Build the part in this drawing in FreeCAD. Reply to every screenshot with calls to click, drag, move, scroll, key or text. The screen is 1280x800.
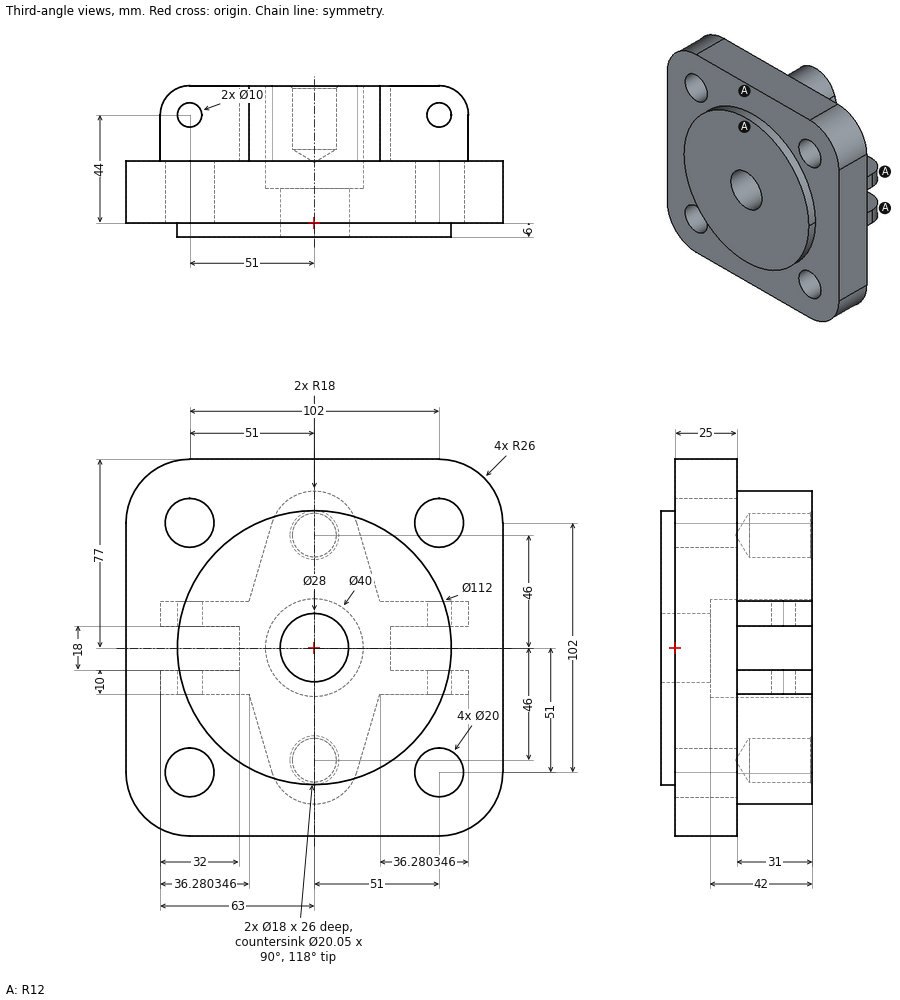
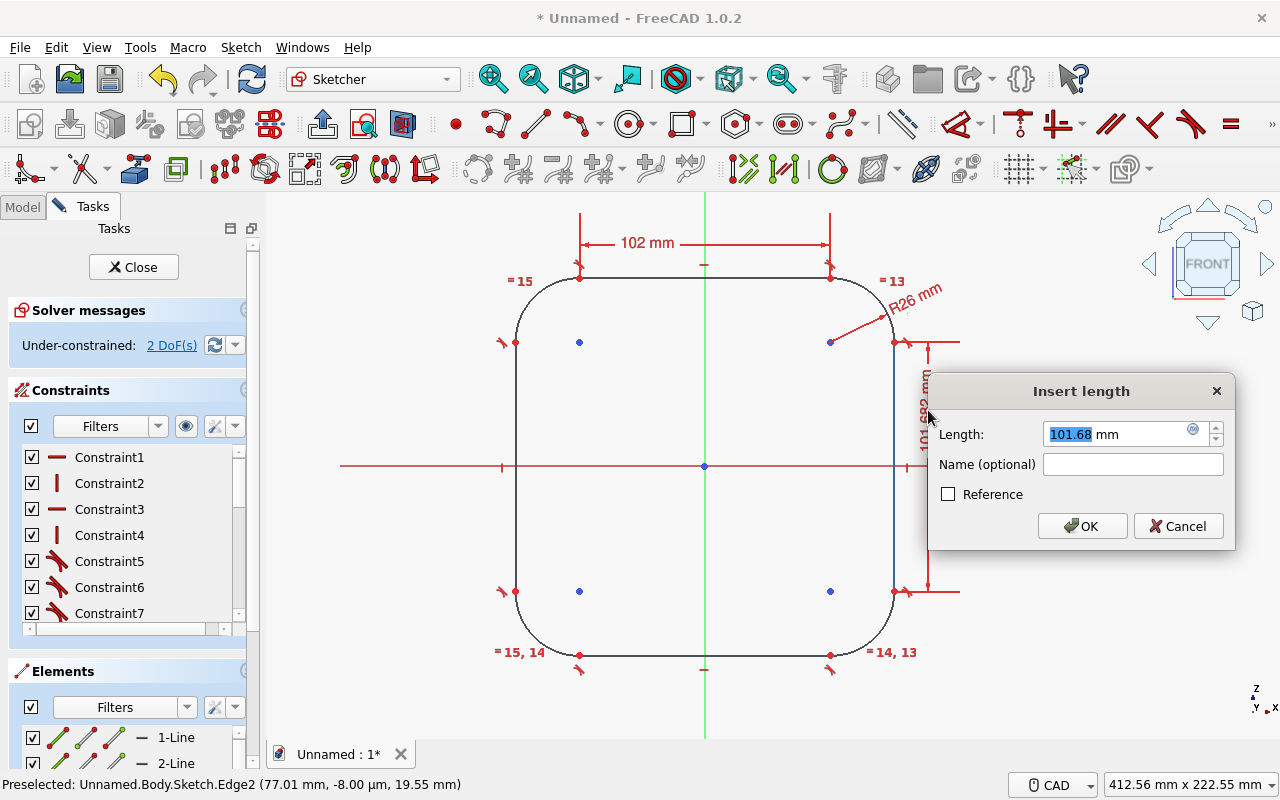
text(102)
key(Return)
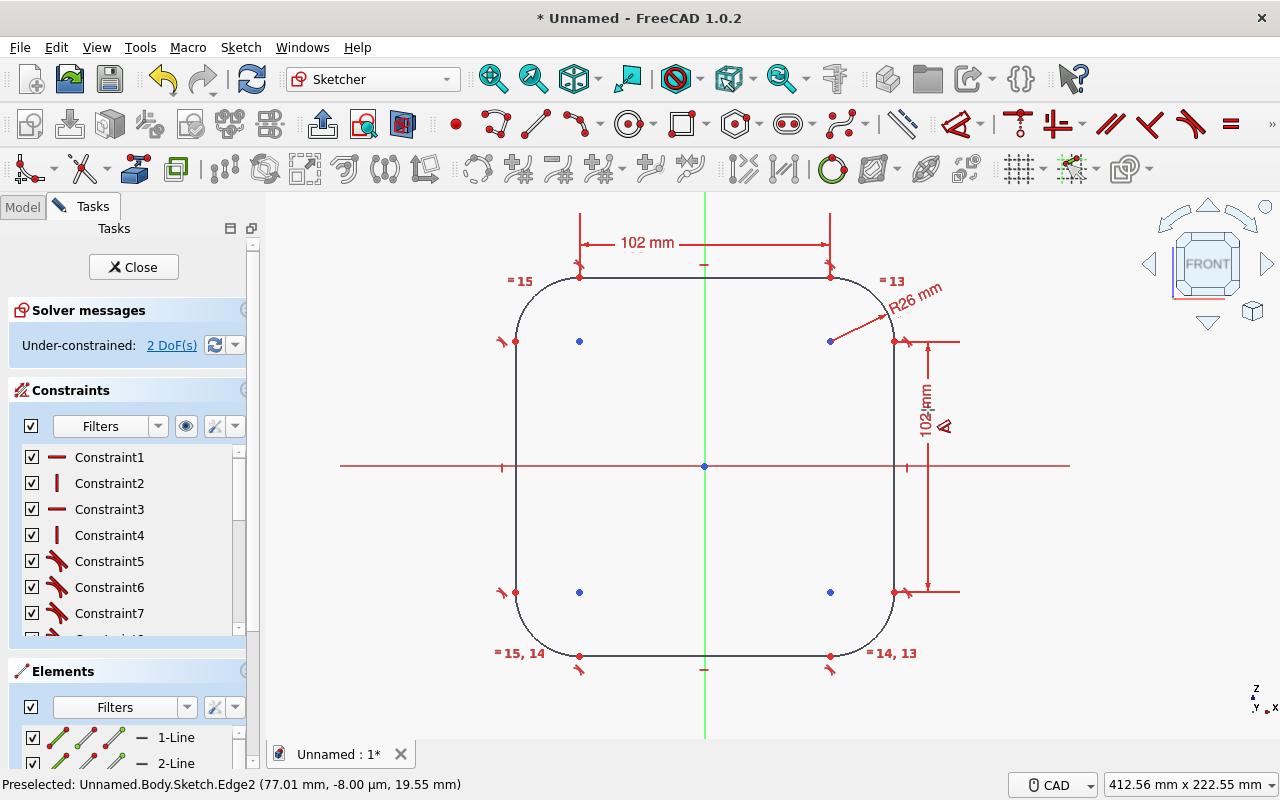
click(580, 278)
click(642, 500)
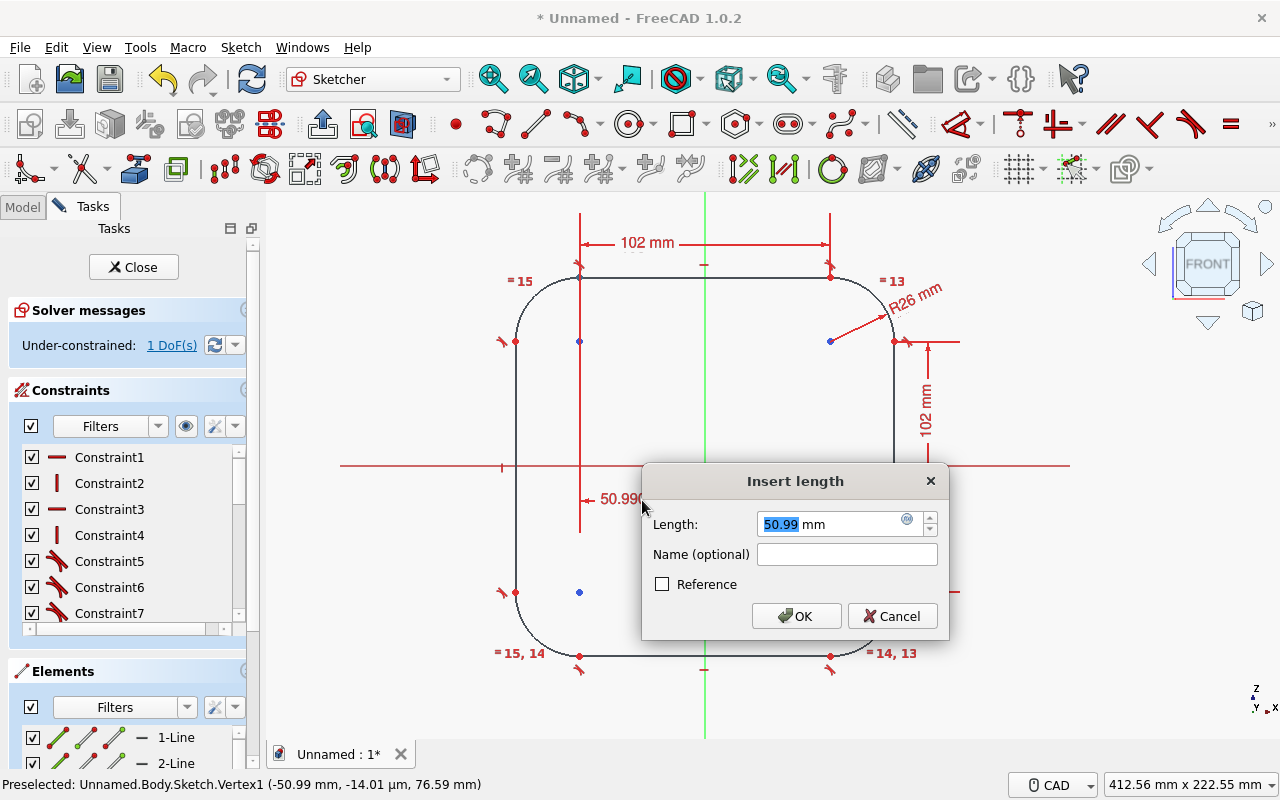
text(51)
key(Return)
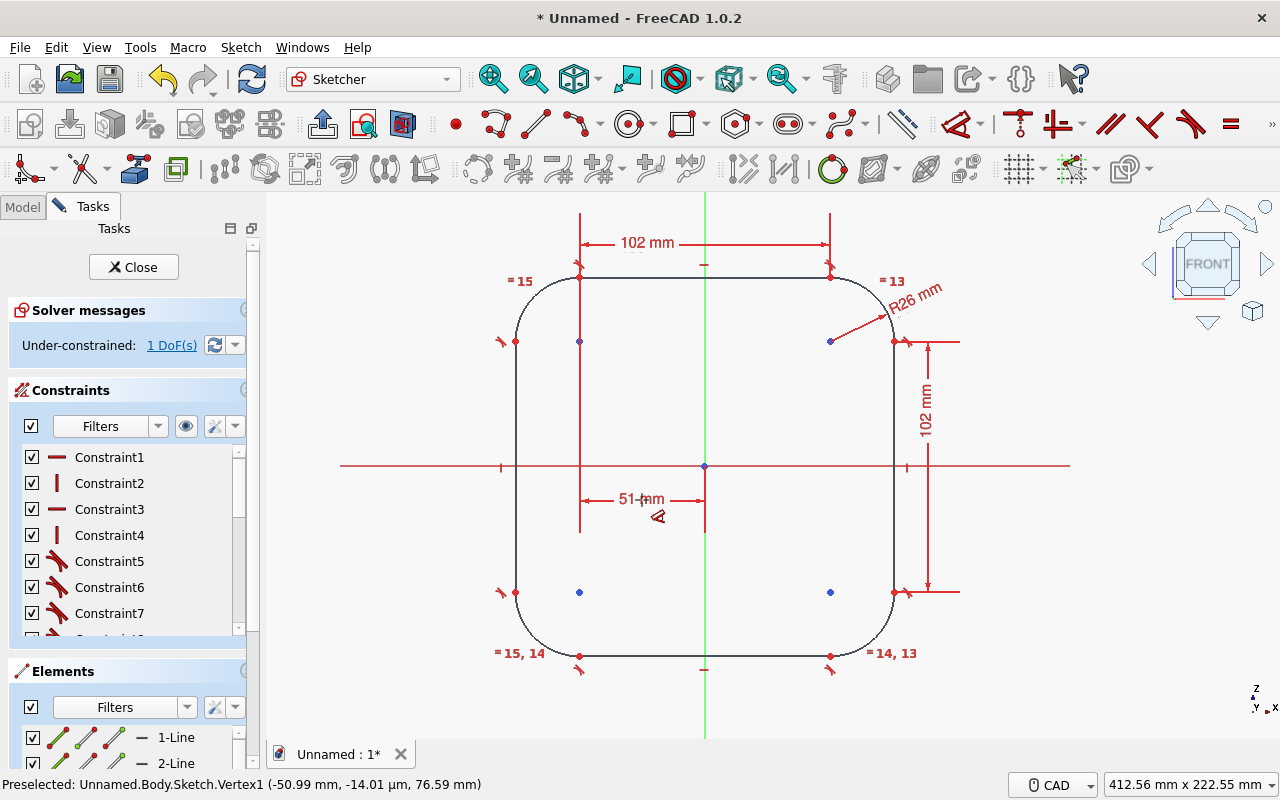
click(580, 278)
click(546, 372)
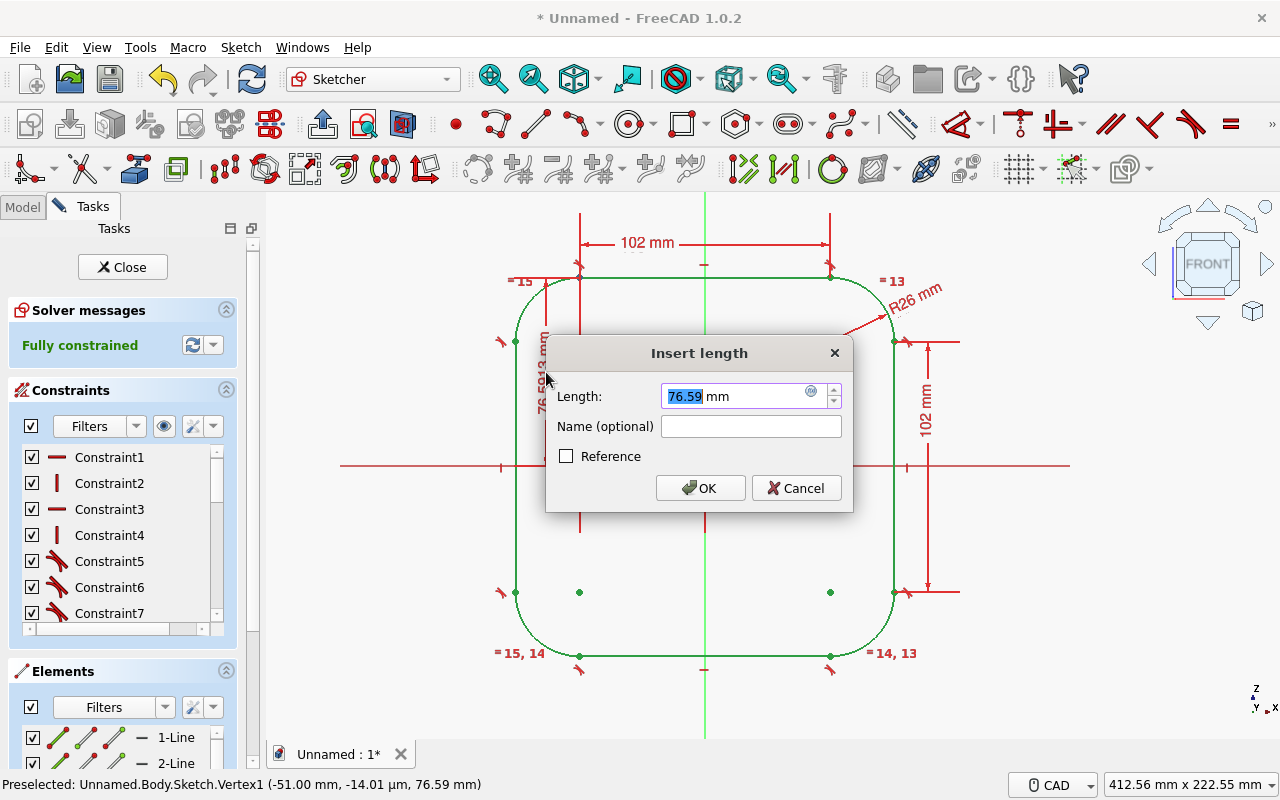
text(77)
key(Return)
key(Escape)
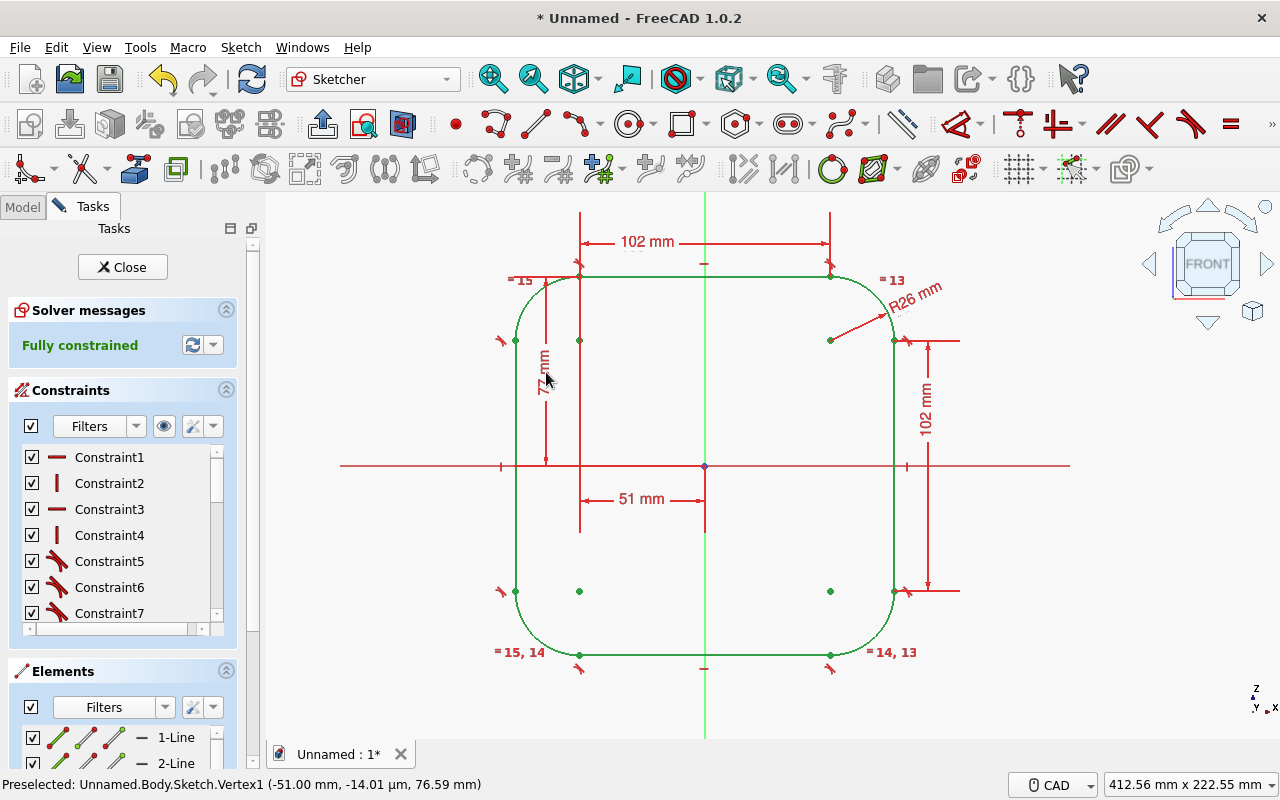
click(123, 267)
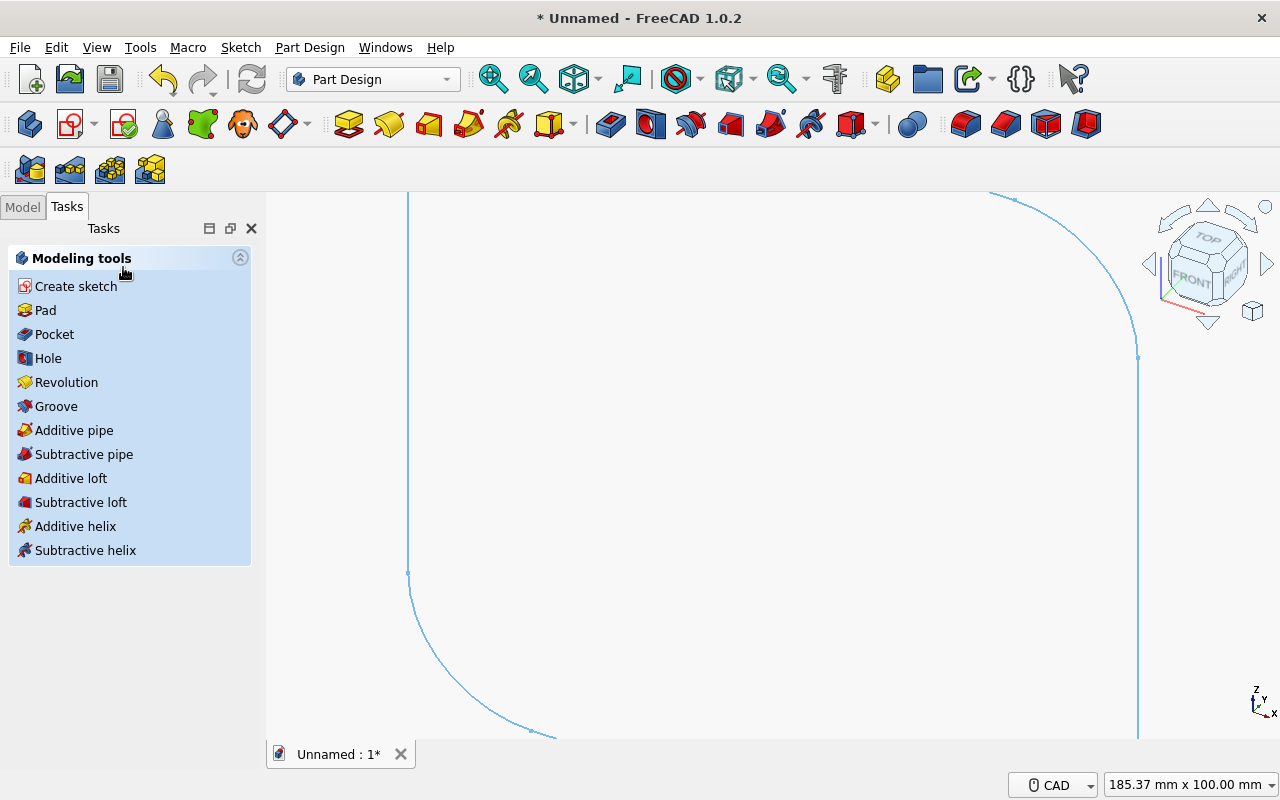
click(350, 124)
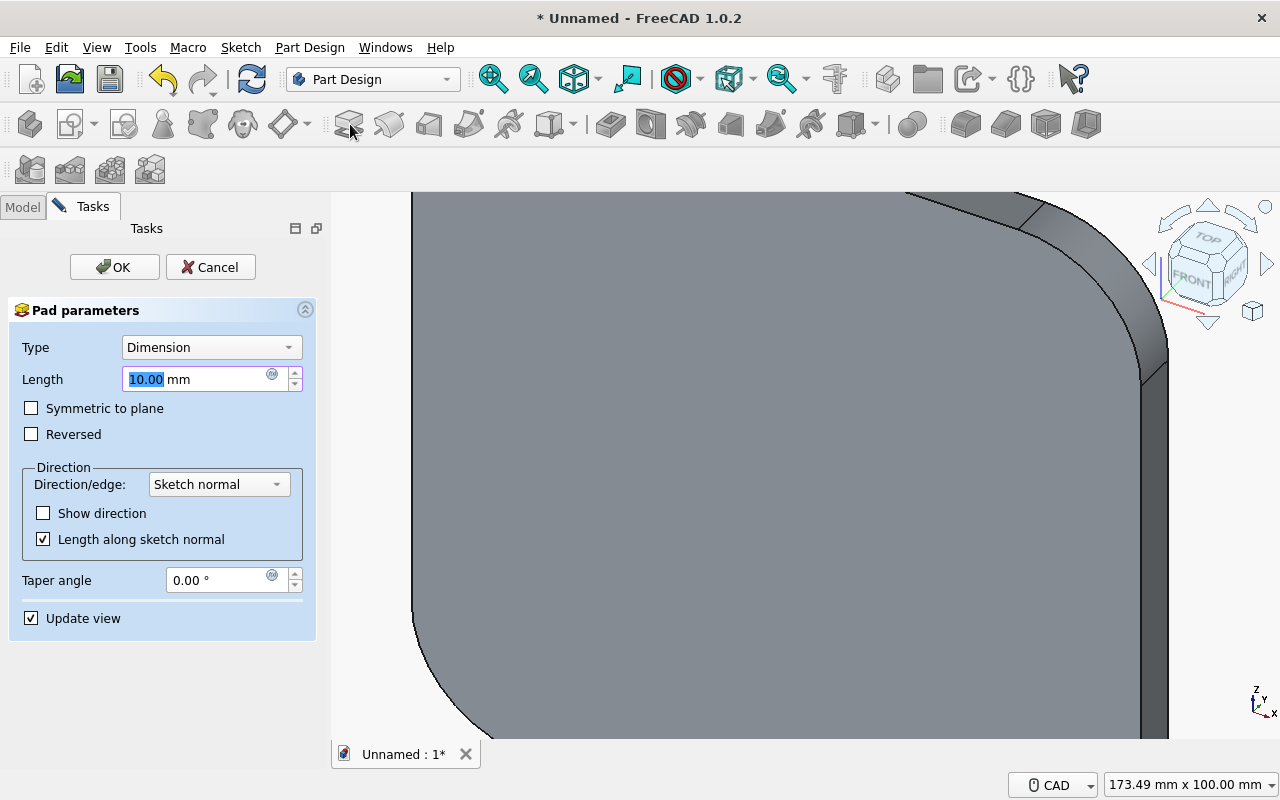
text(25)
key(Tab)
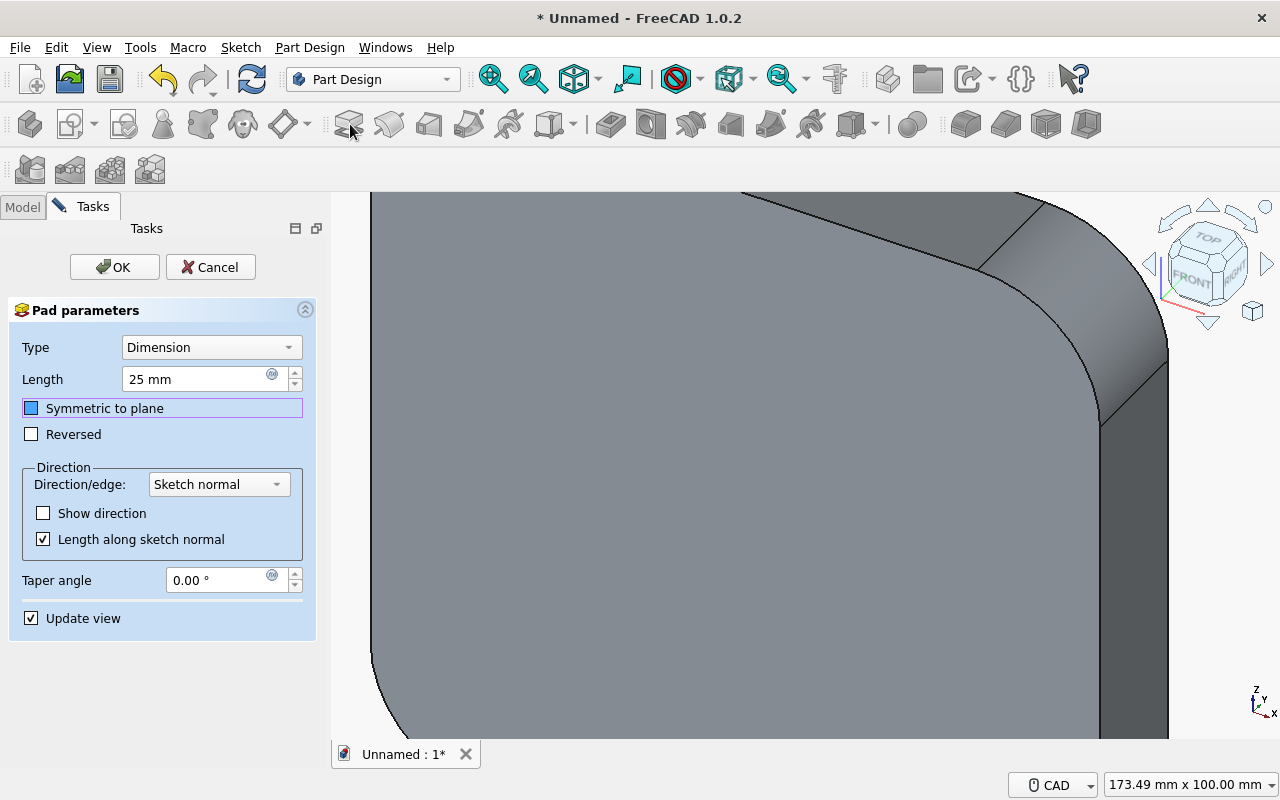
click(30, 434)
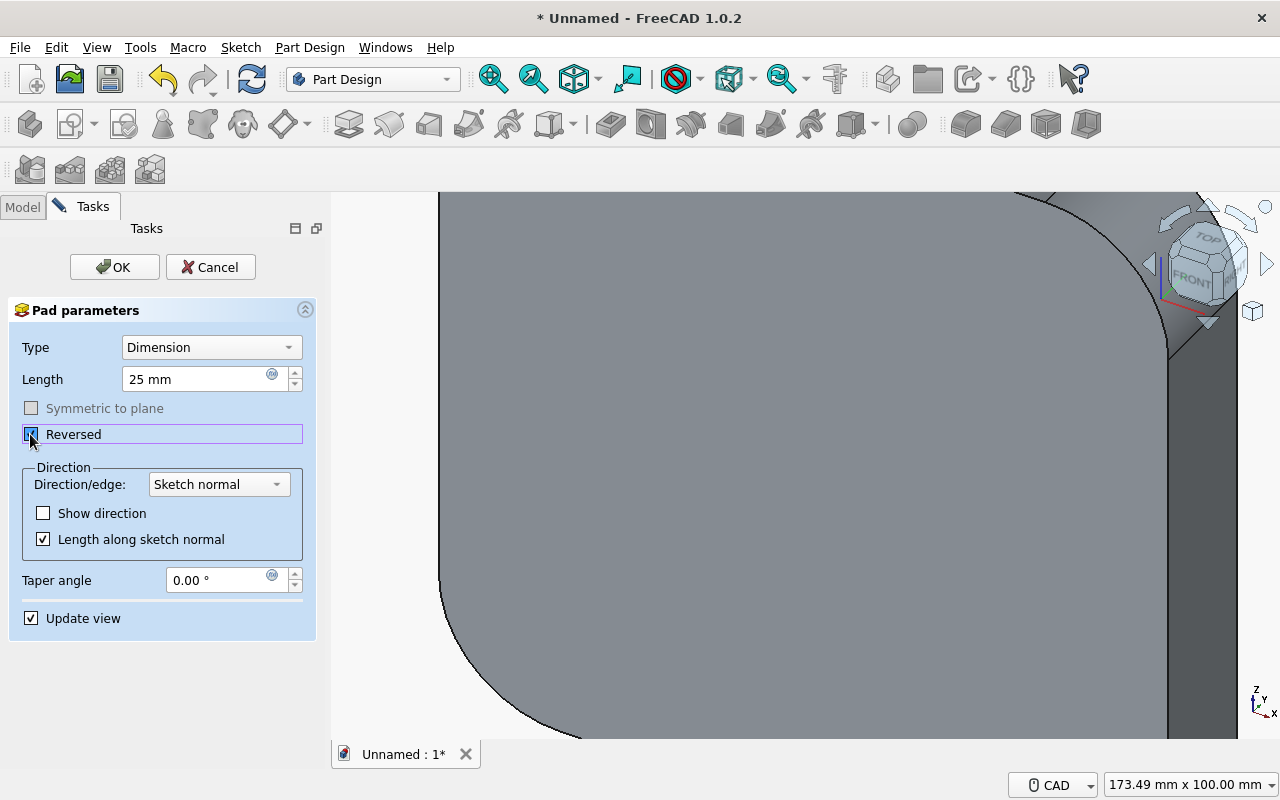
click(115, 267)